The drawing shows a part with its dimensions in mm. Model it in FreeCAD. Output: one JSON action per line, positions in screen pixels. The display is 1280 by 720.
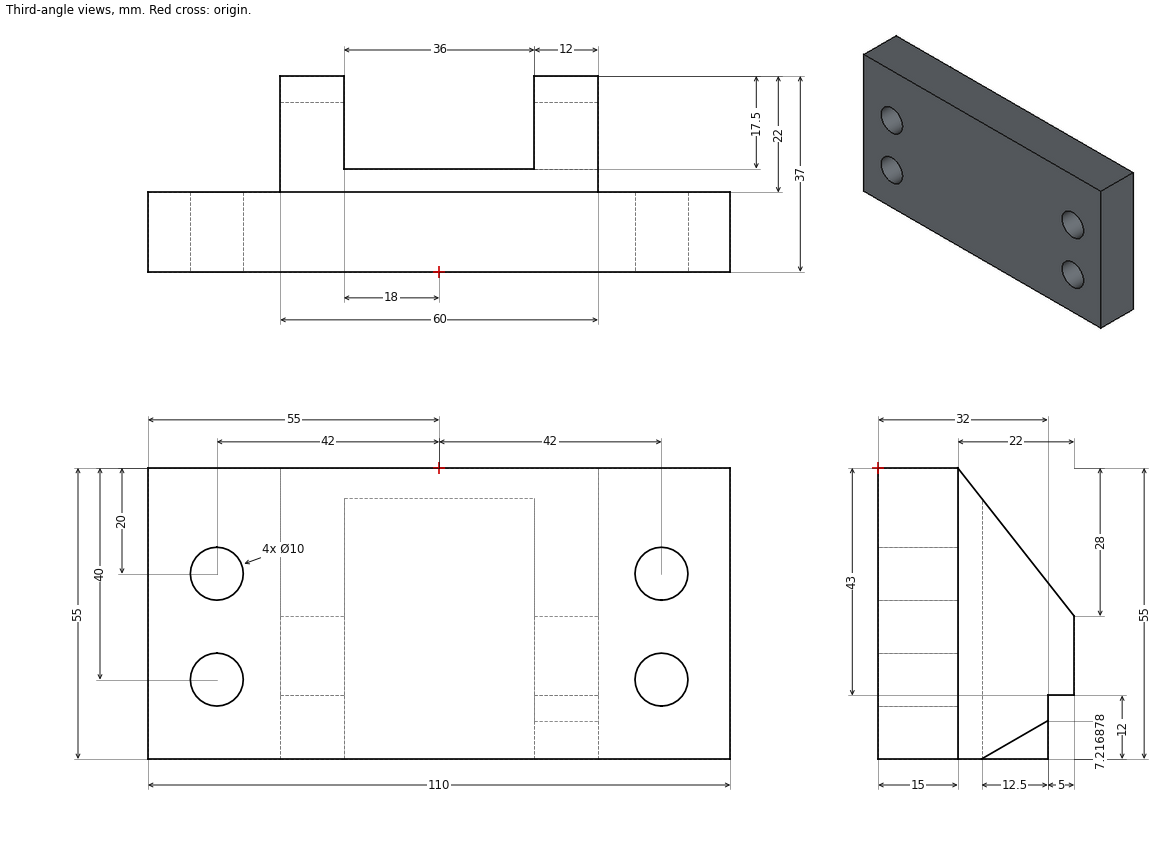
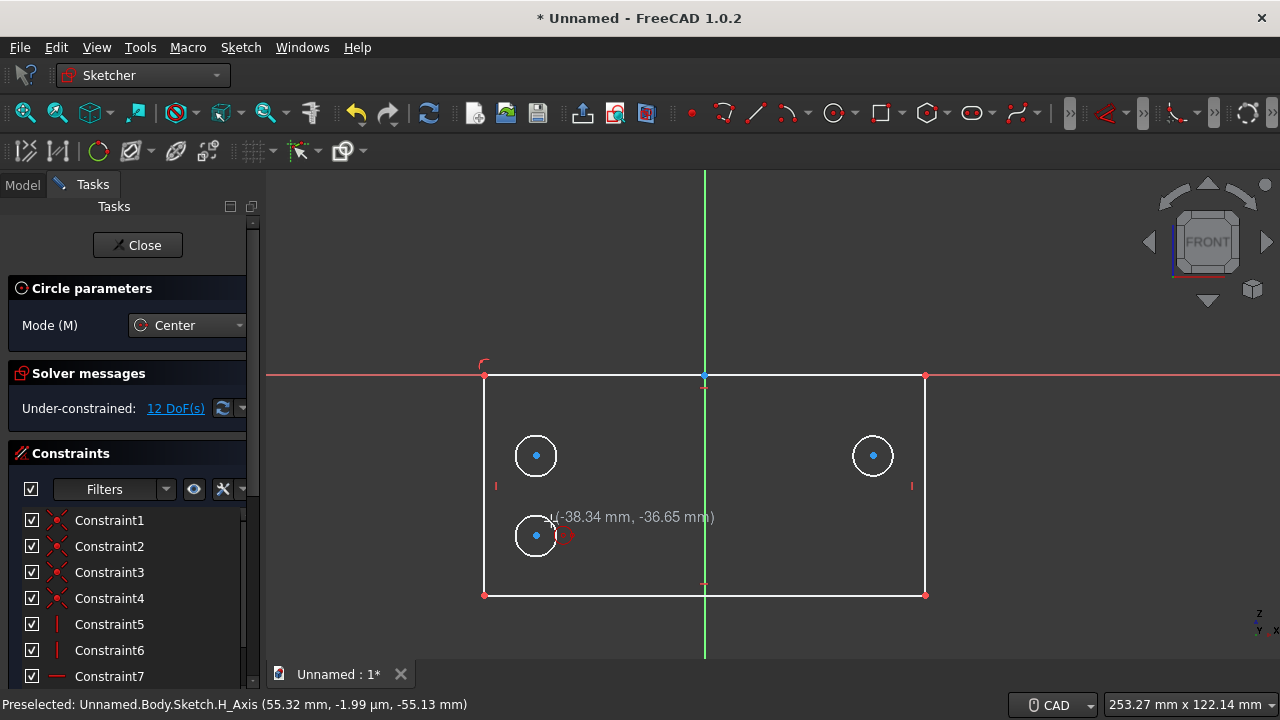
{"action": "left_click", "coordinate": [873, 535]}
{"action": "left_click", "coordinate": [887, 521]}
{"action": "key", "text": "Escape"}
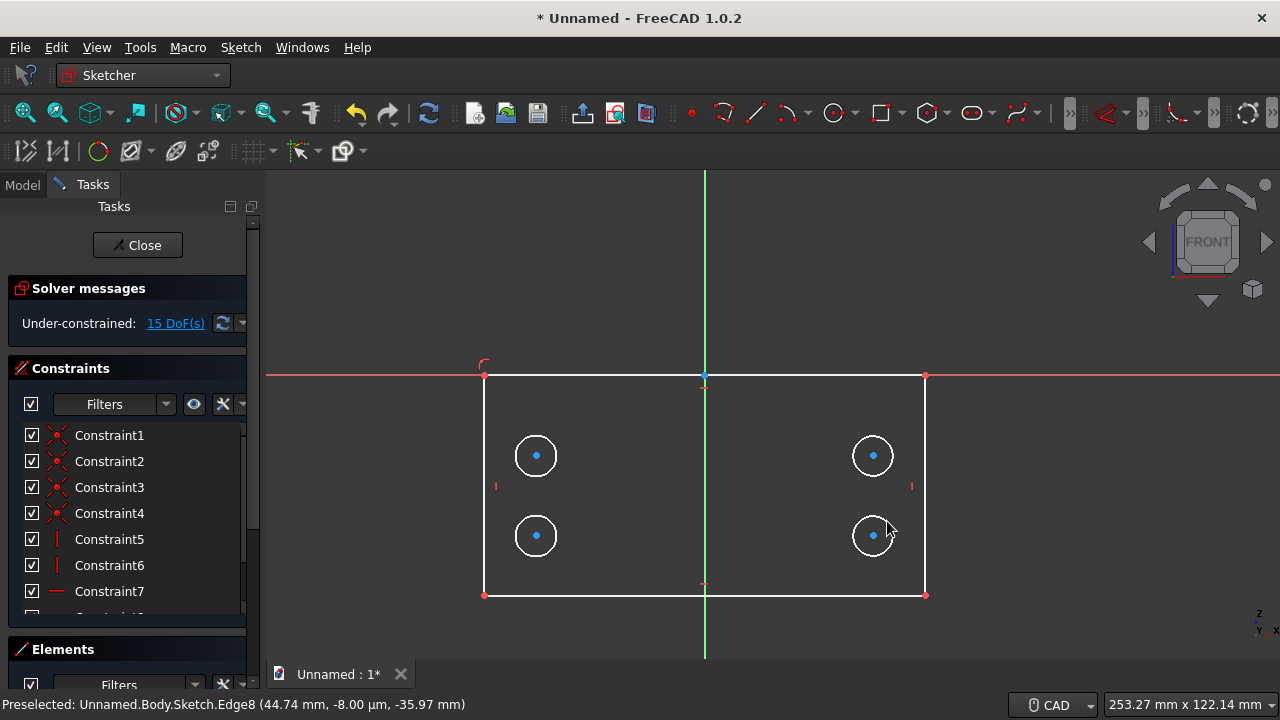
{"action": "left_click", "coordinate": [550, 441]}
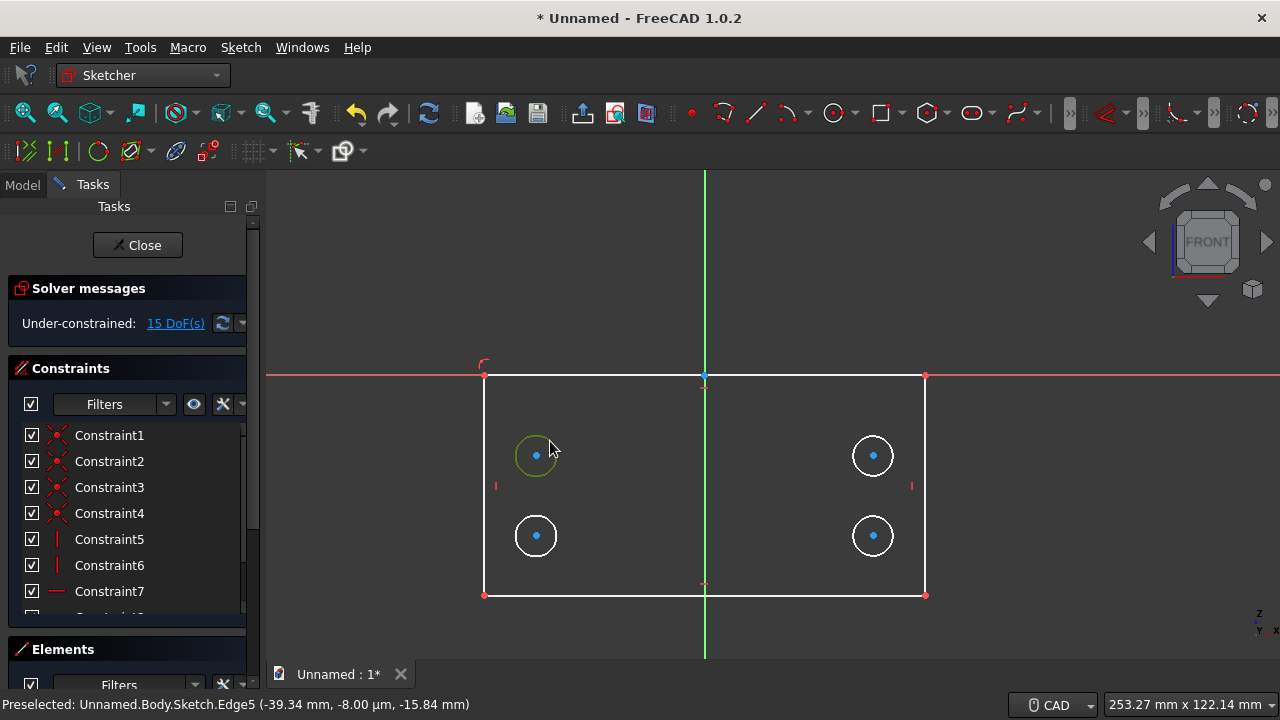
{"action": "left_click", "coordinate": [887, 442]}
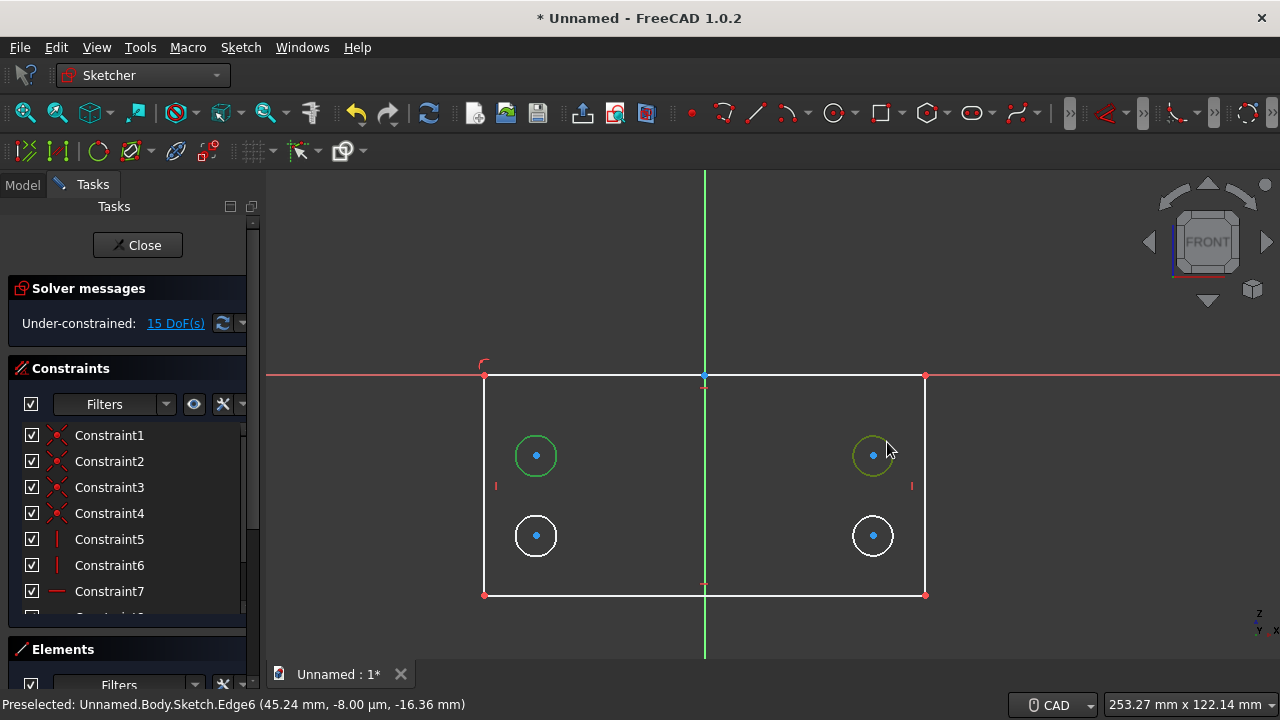
{"action": "left_click", "coordinate": [550, 521]}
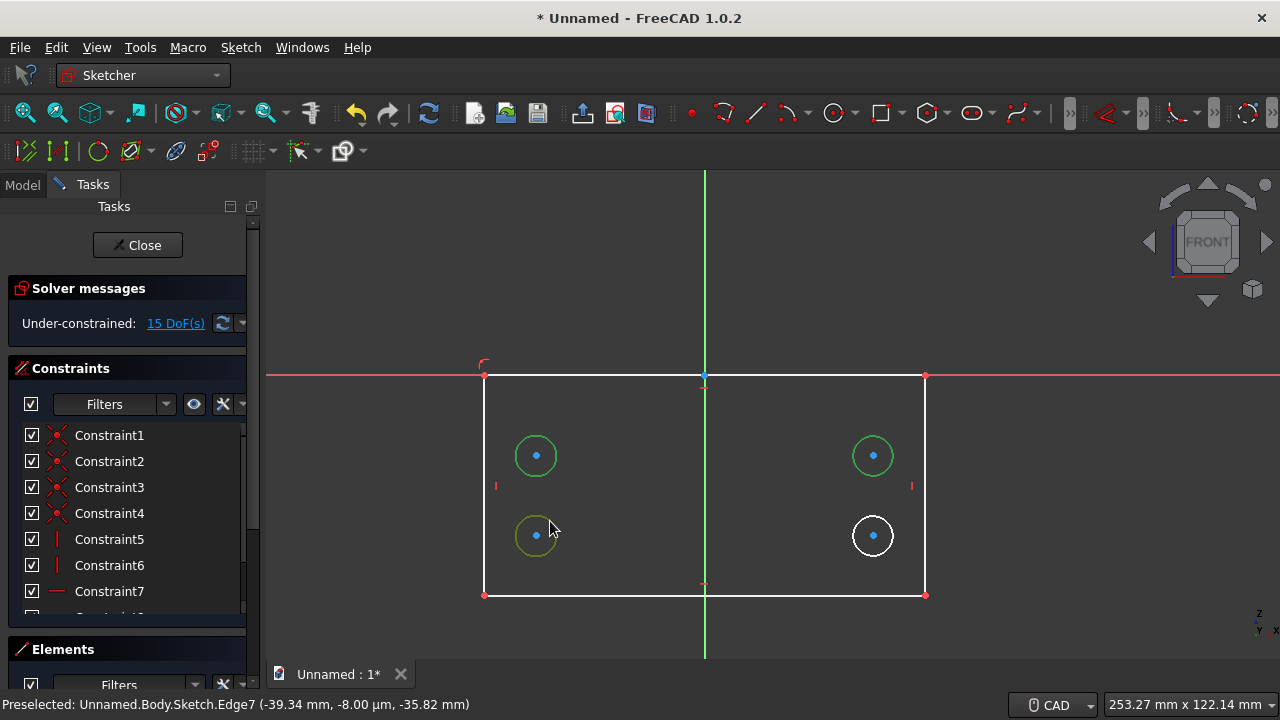
{"action": "left_click", "coordinate": [887, 522]}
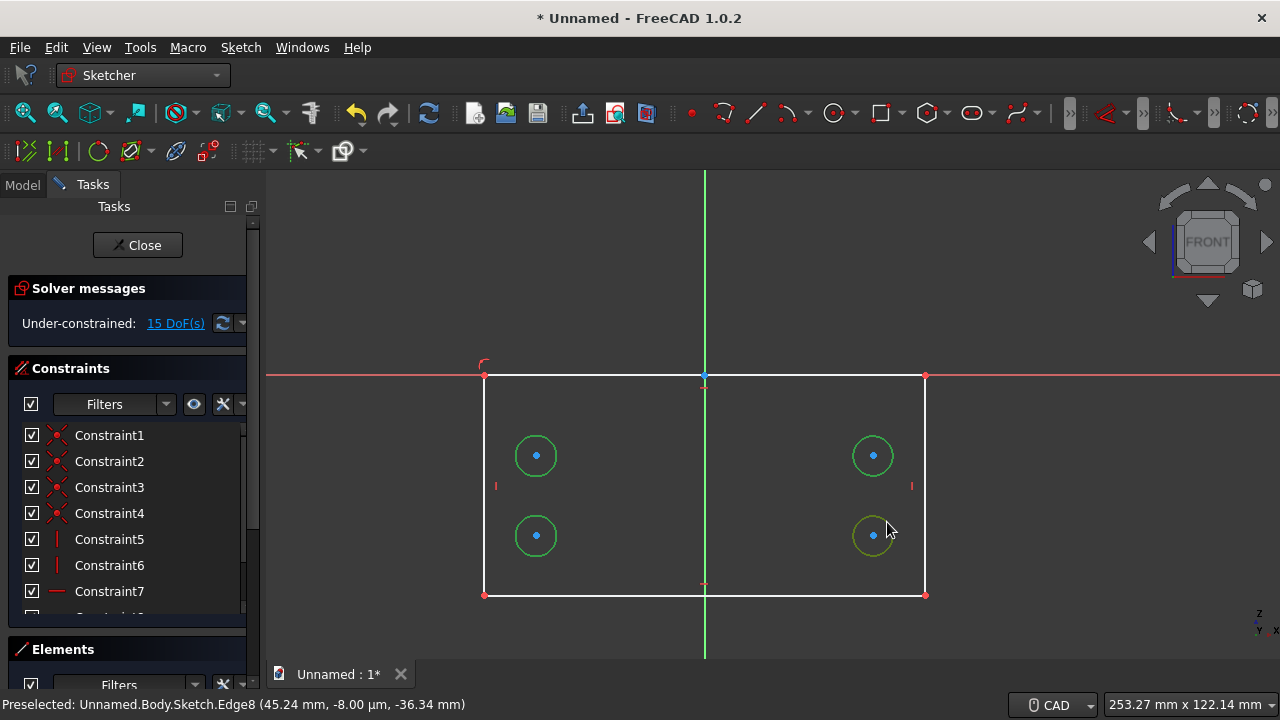
{"action": "key", "text": "e"}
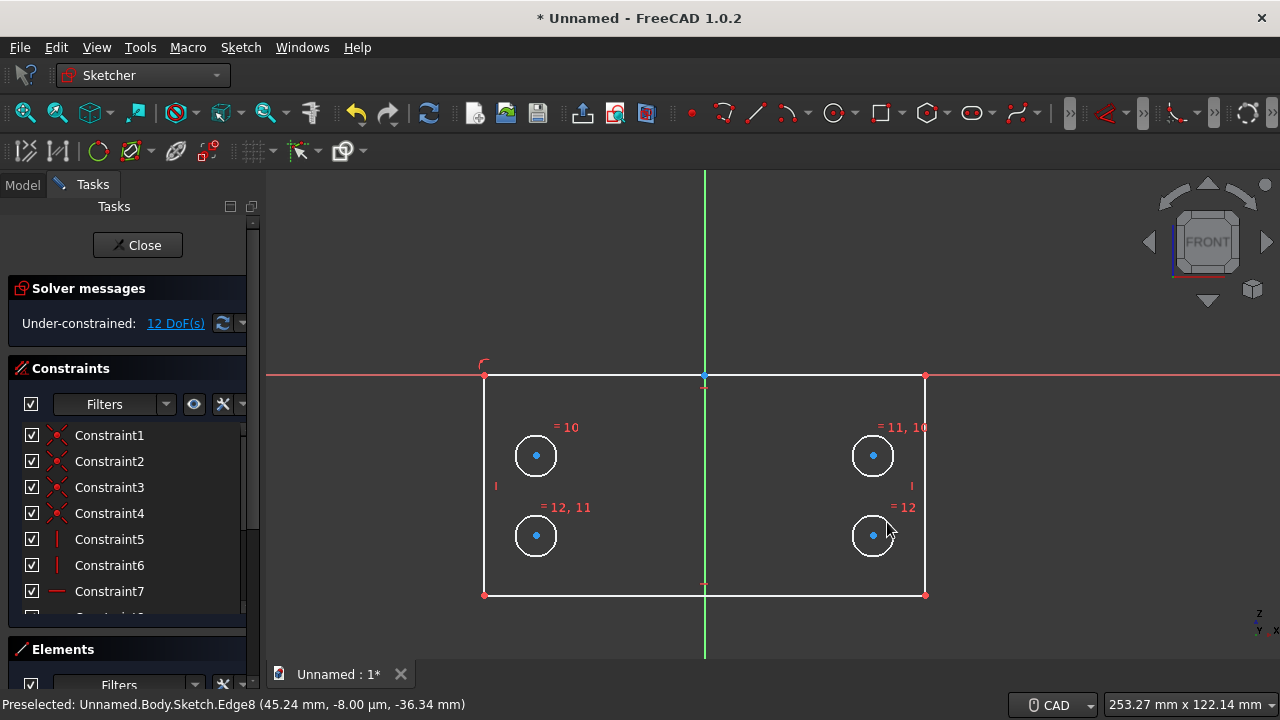
{"action": "left_click", "coordinate": [550, 441]}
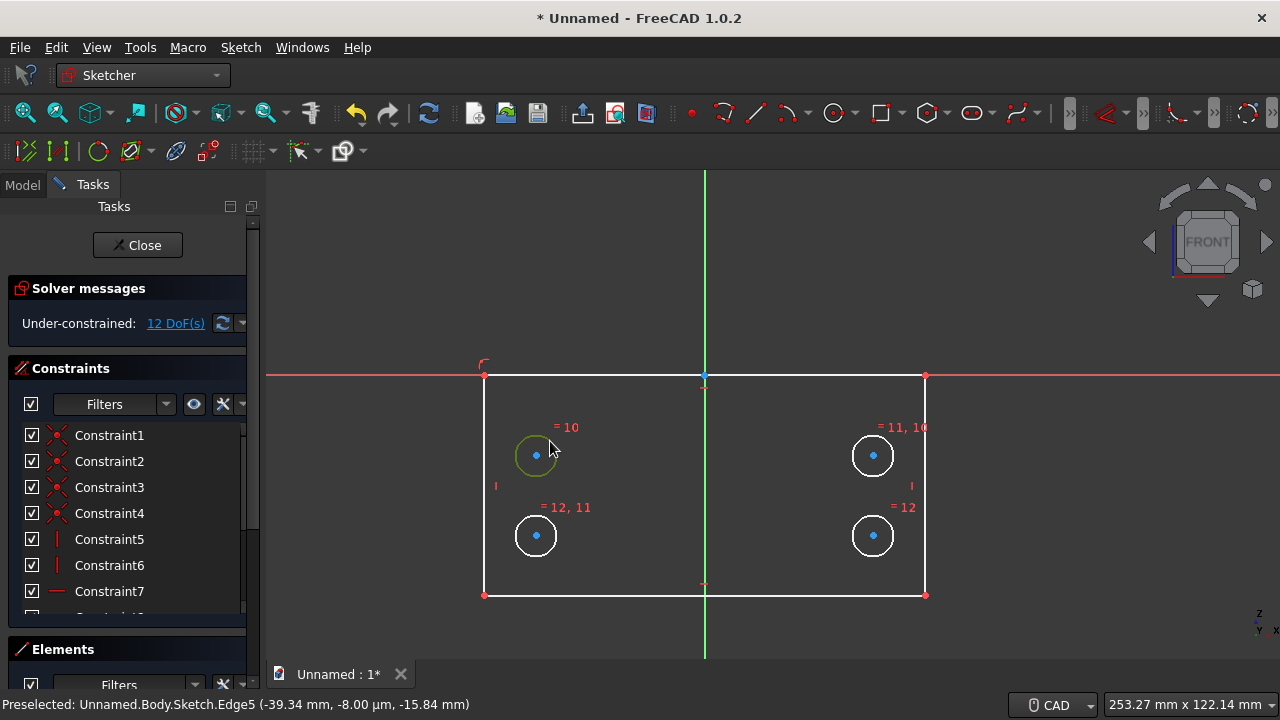
{"action": "left_click", "coordinate": [1128, 114]}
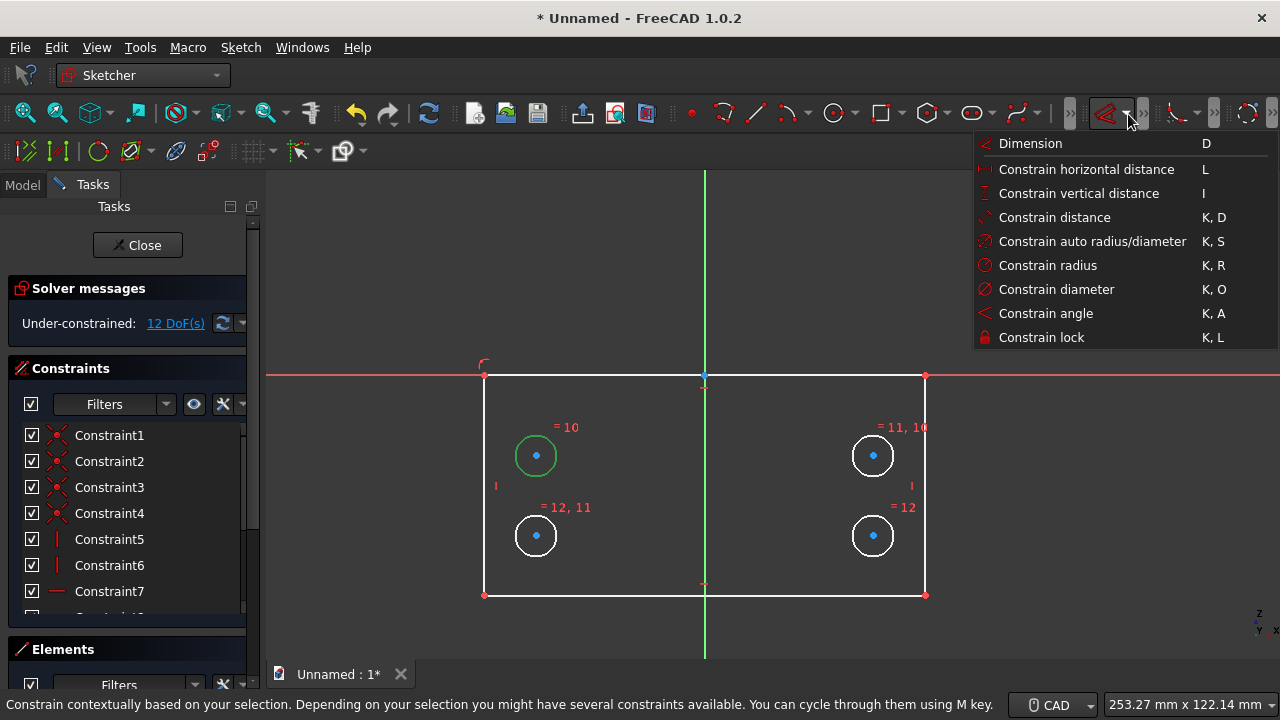
{"action": "left_click", "coordinate": [1126, 289]}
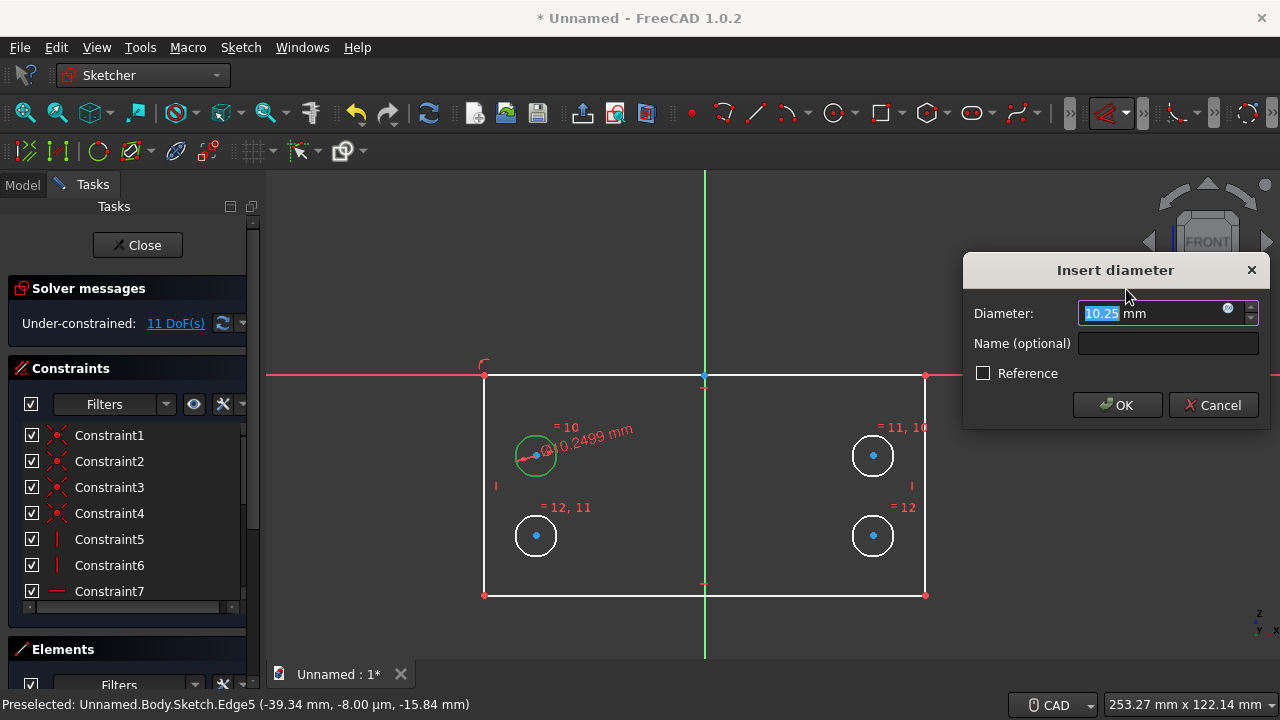
{"action": "type", "text": "10"}
{"action": "key", "text": "Return"}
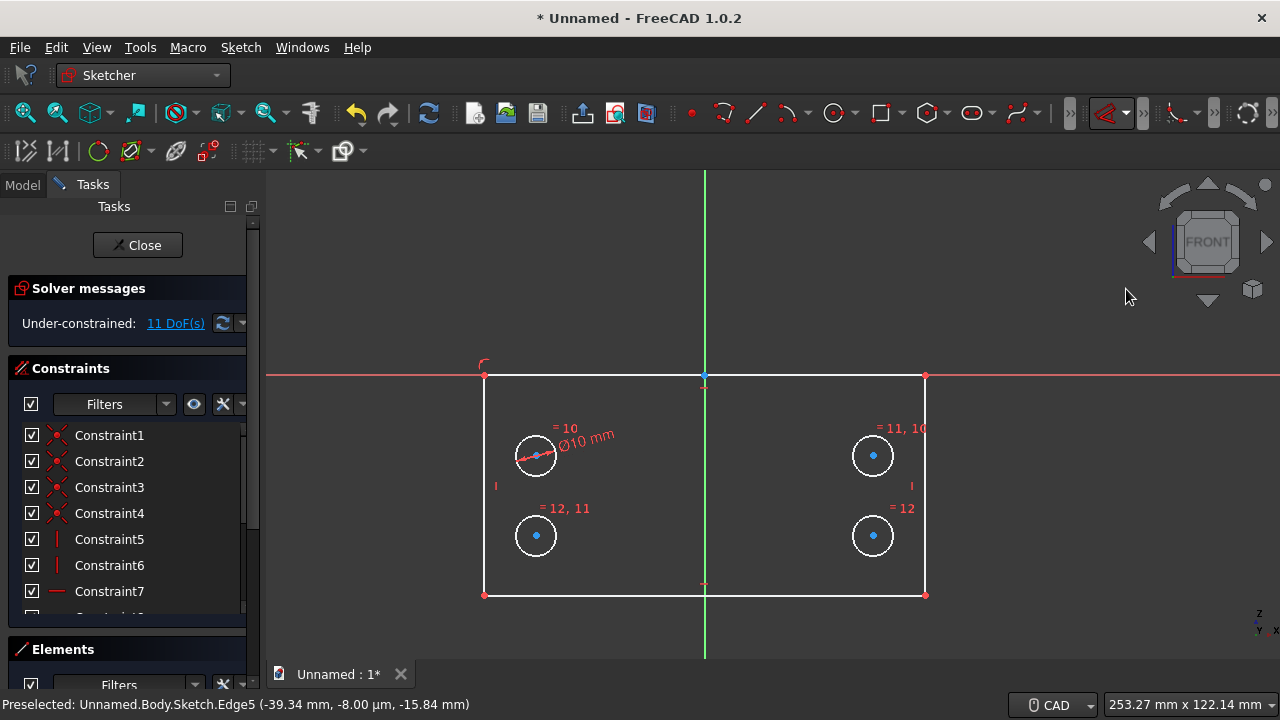
{"action": "left_click", "coordinate": [484, 441]}